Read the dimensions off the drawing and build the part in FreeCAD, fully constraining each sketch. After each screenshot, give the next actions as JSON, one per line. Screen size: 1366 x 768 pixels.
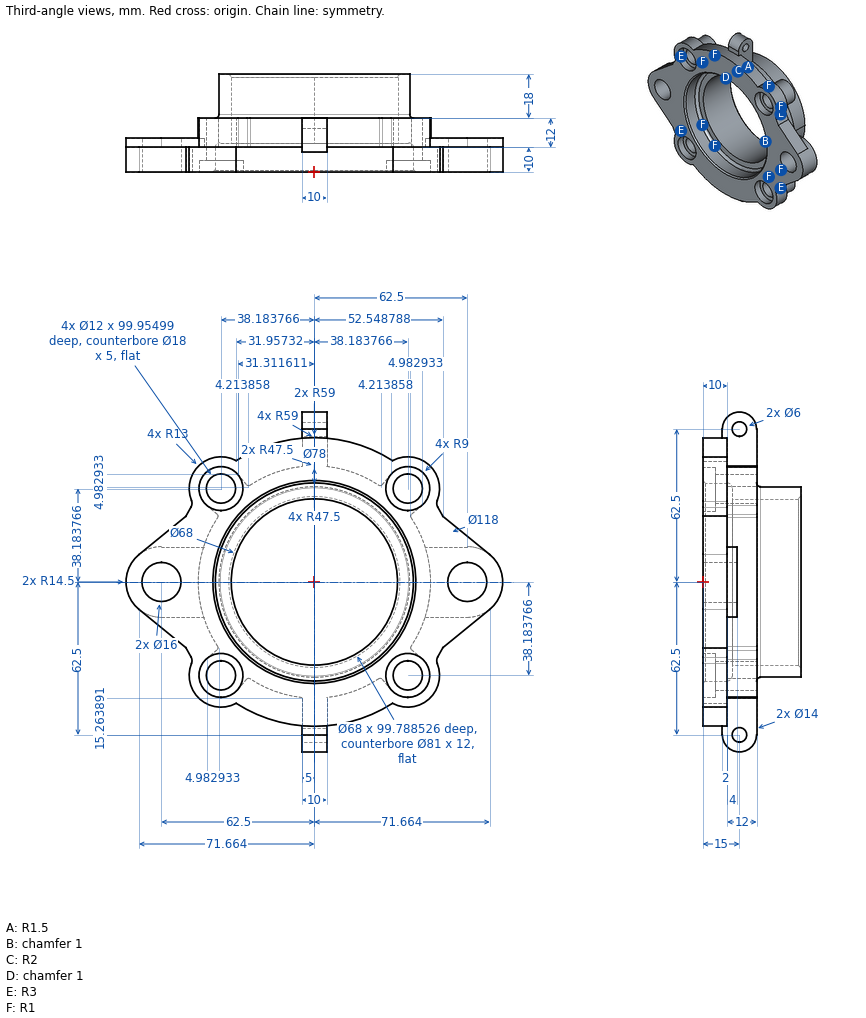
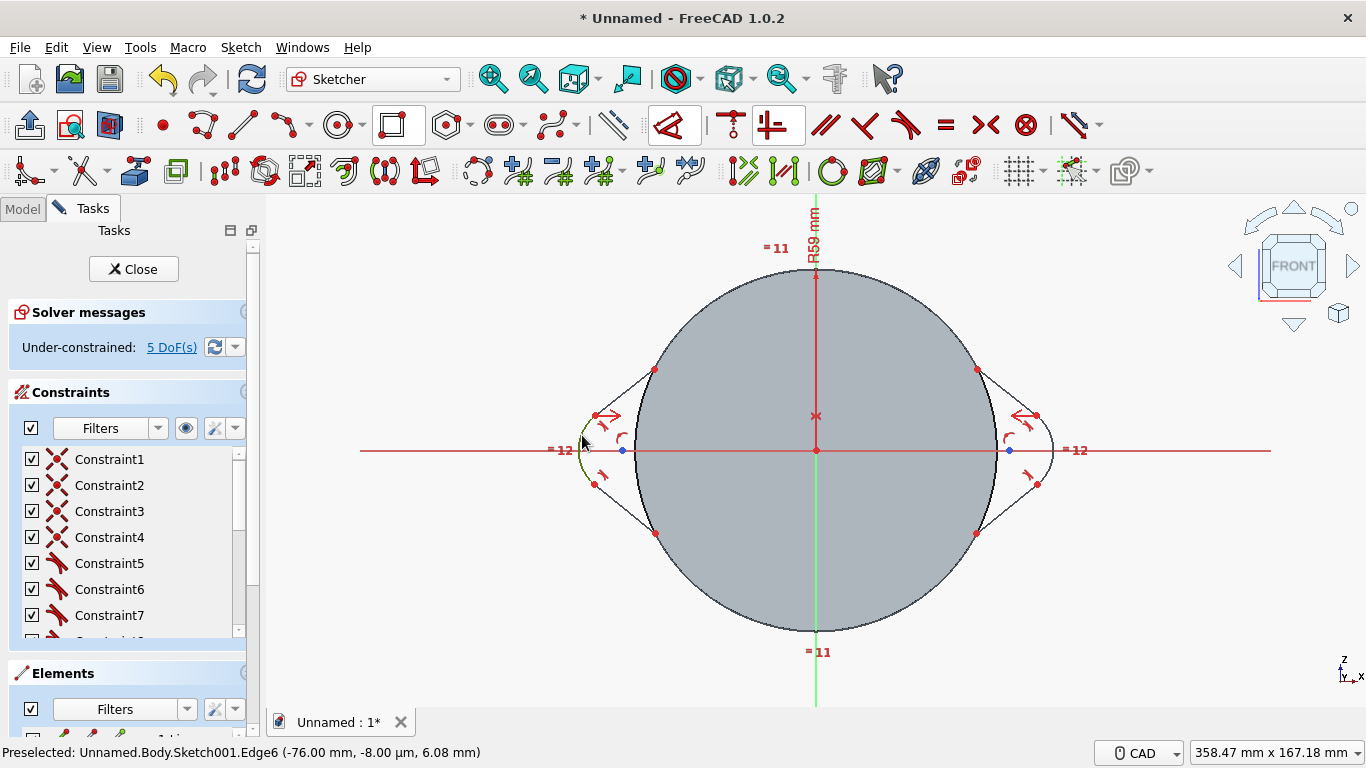
{"action": "left_click", "coordinate": [696, 126]}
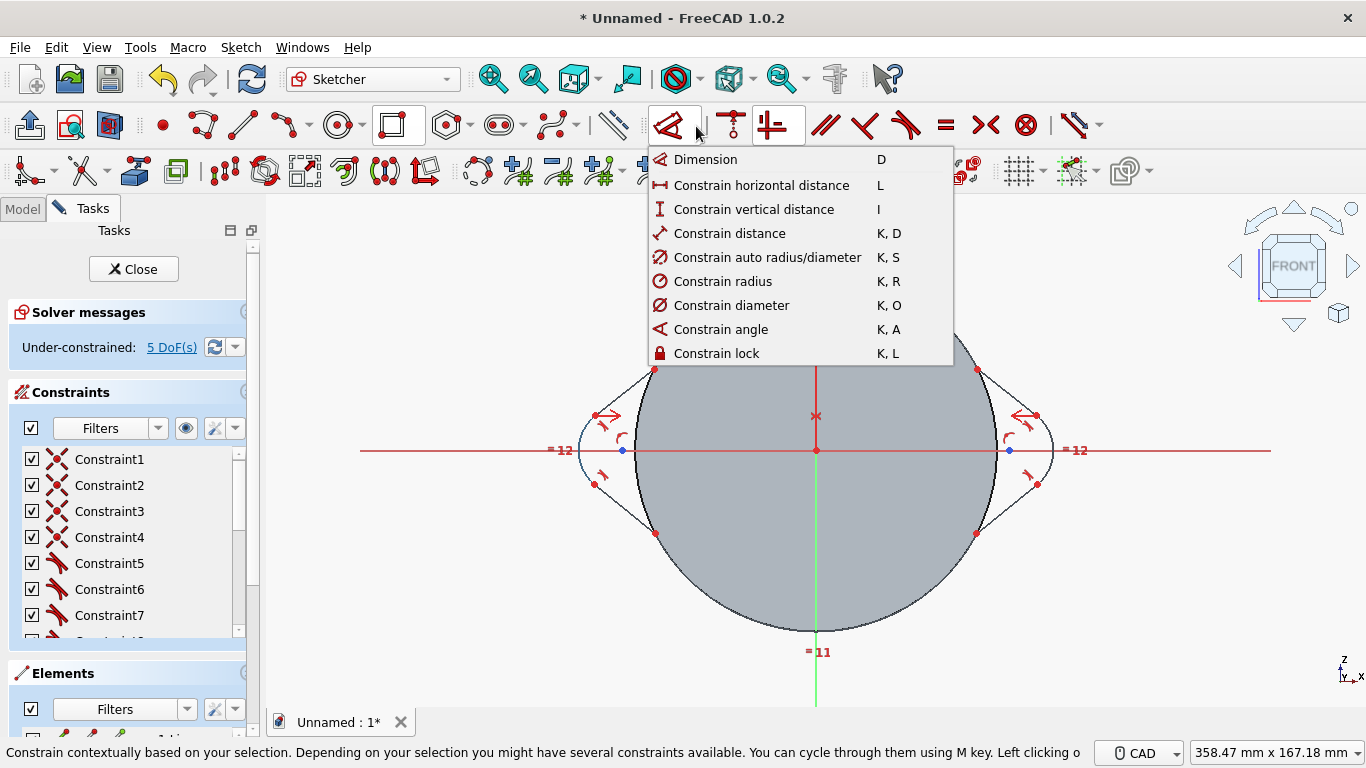
{"action": "left_click", "coordinate": [801, 281]}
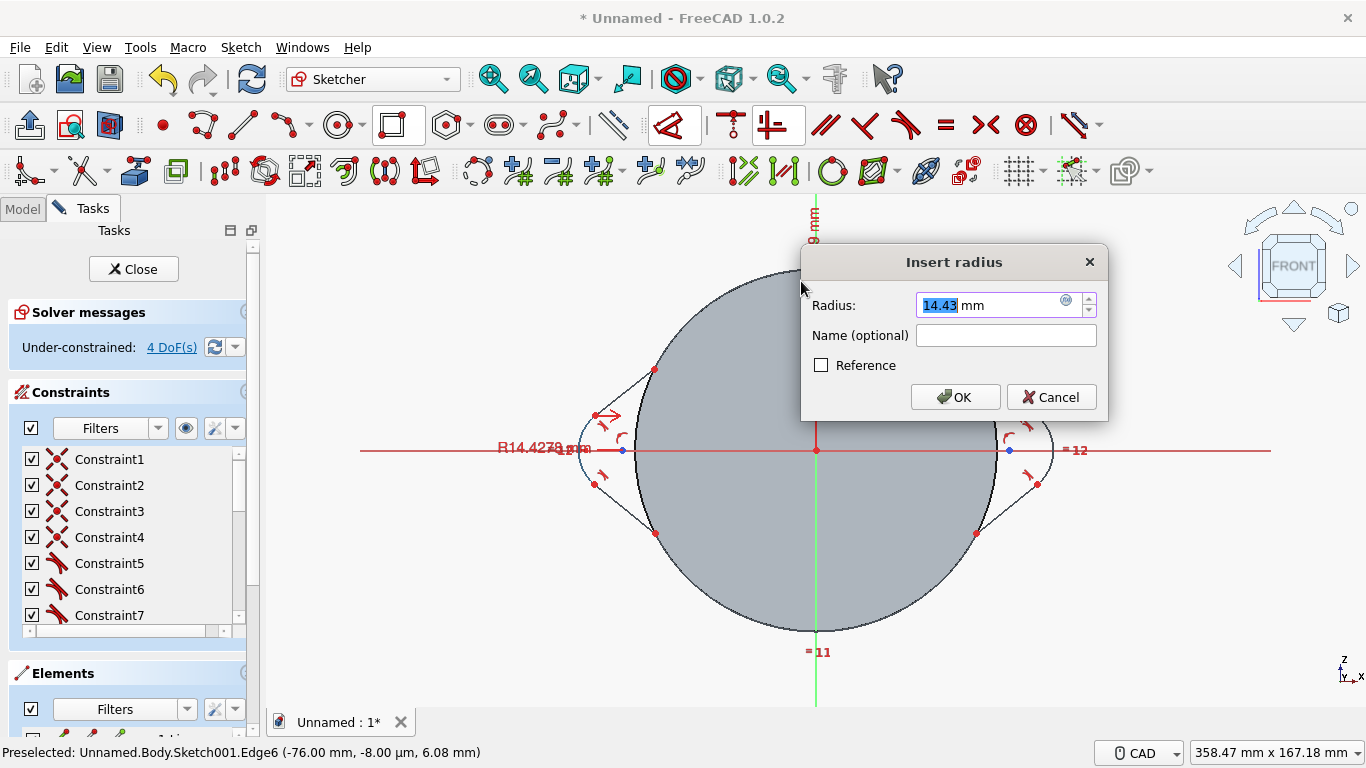
{"action": "type", "text": "14.5"}
{"action": "key", "text": "Return"}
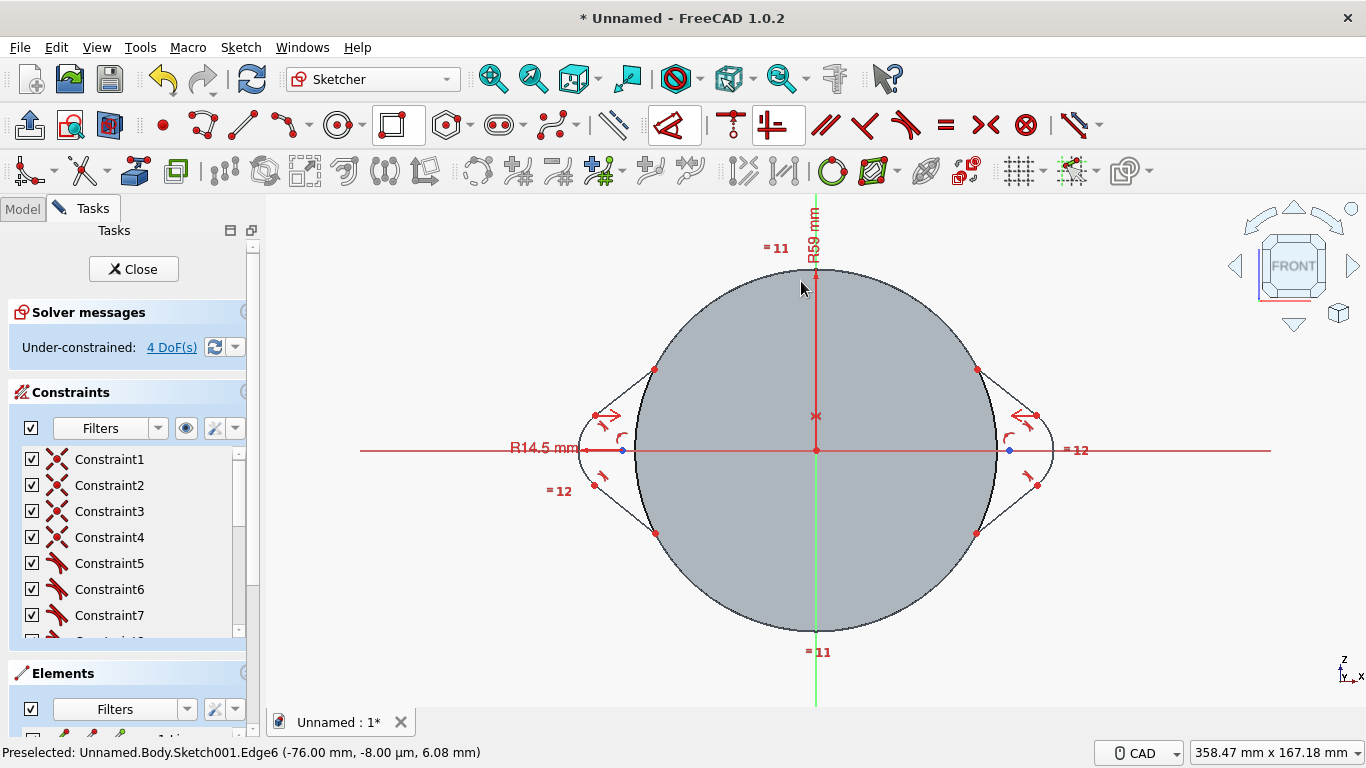
{"action": "left_click", "coordinate": [623, 450]}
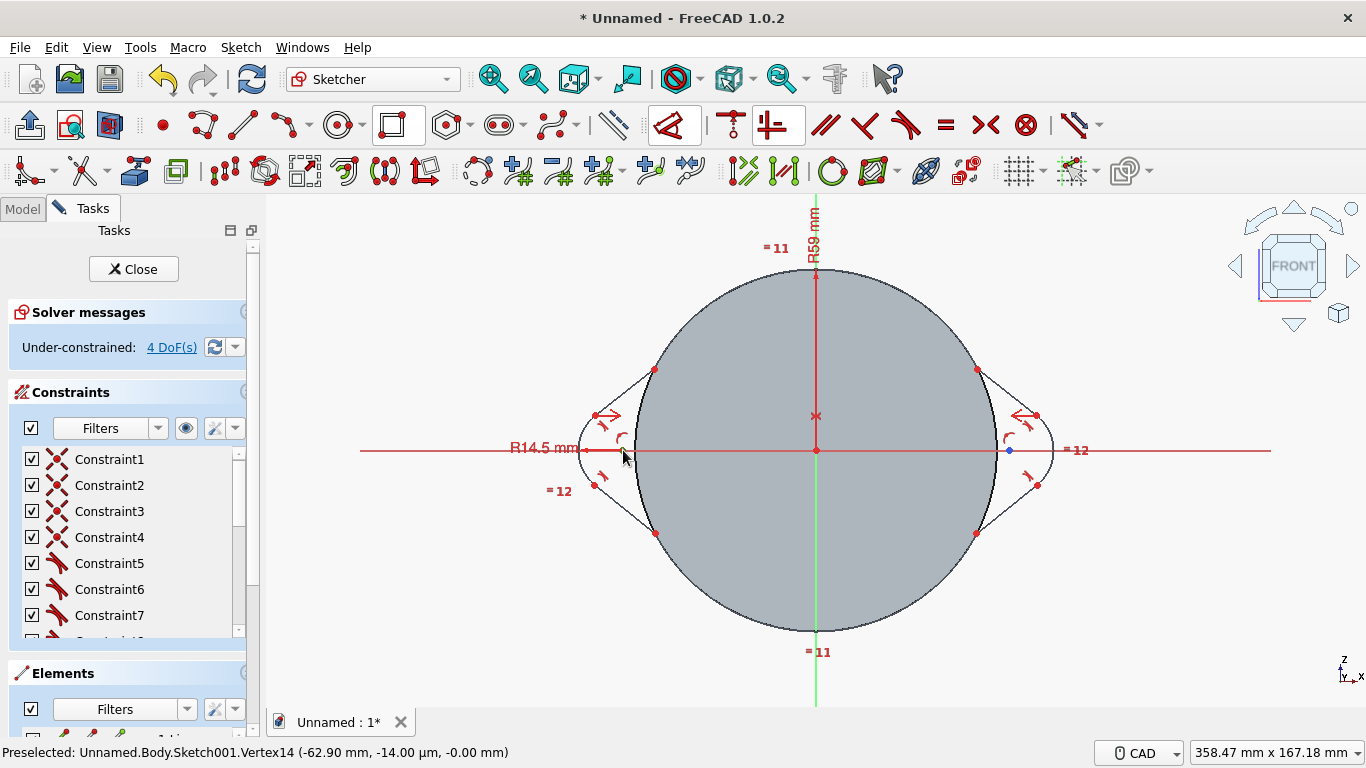
{"action": "left_click", "coordinate": [696, 126]}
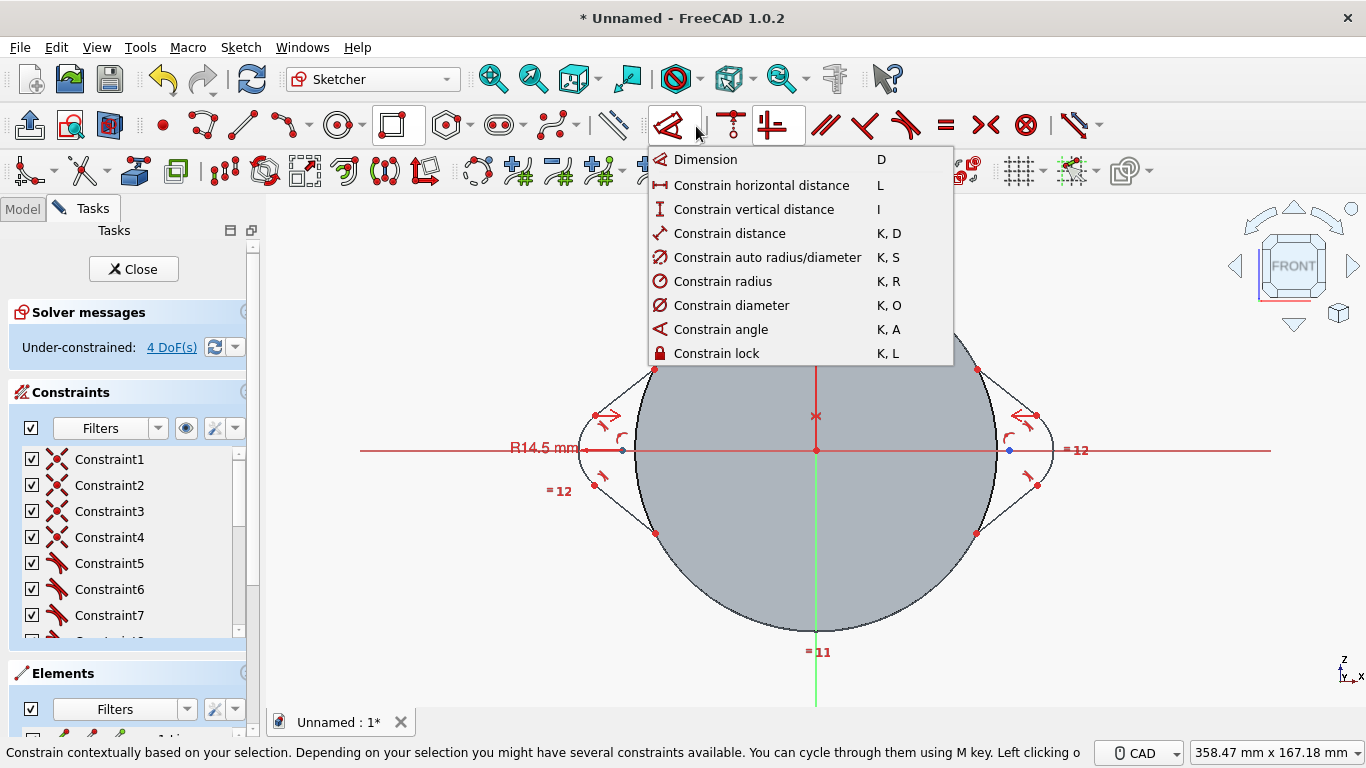
{"action": "left_click", "coordinate": [801, 185]}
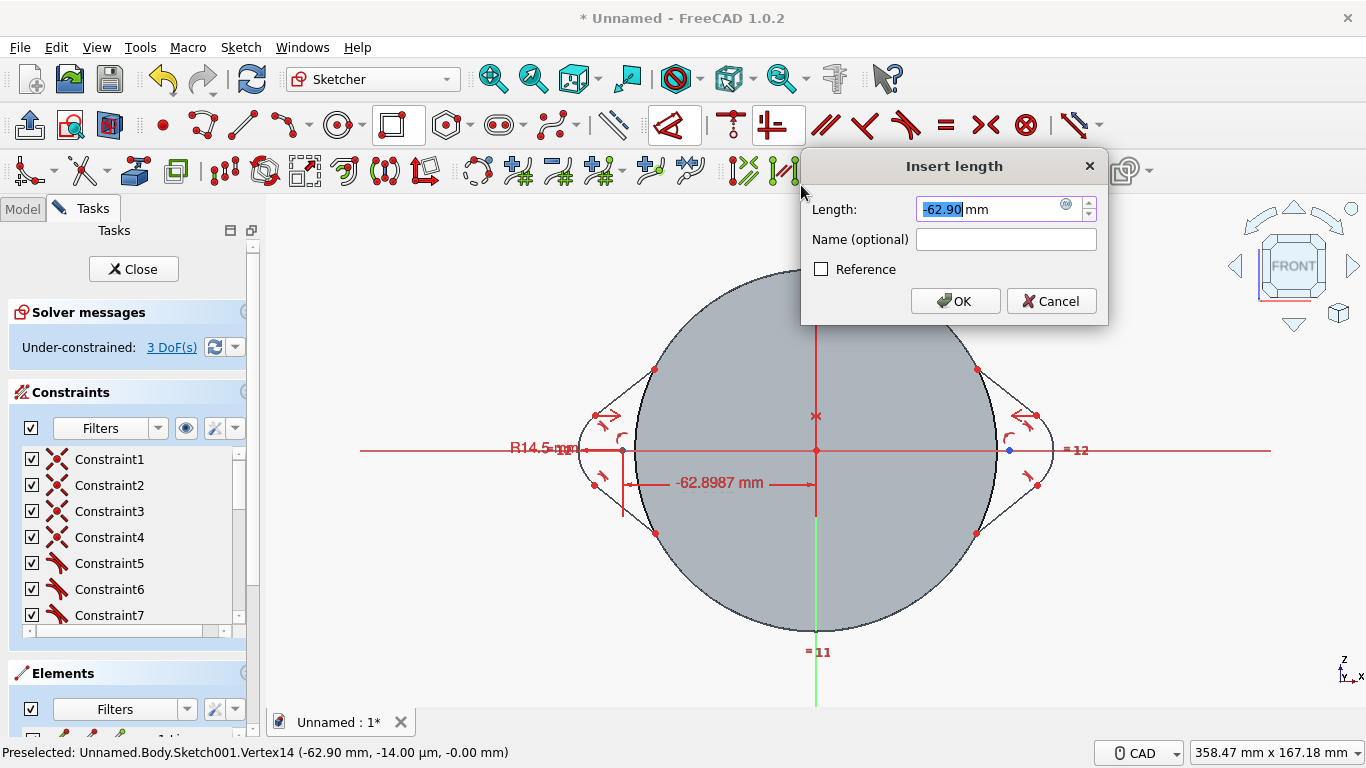
{"action": "type", "text": "-62.5"}
{"action": "key", "text": "Return"}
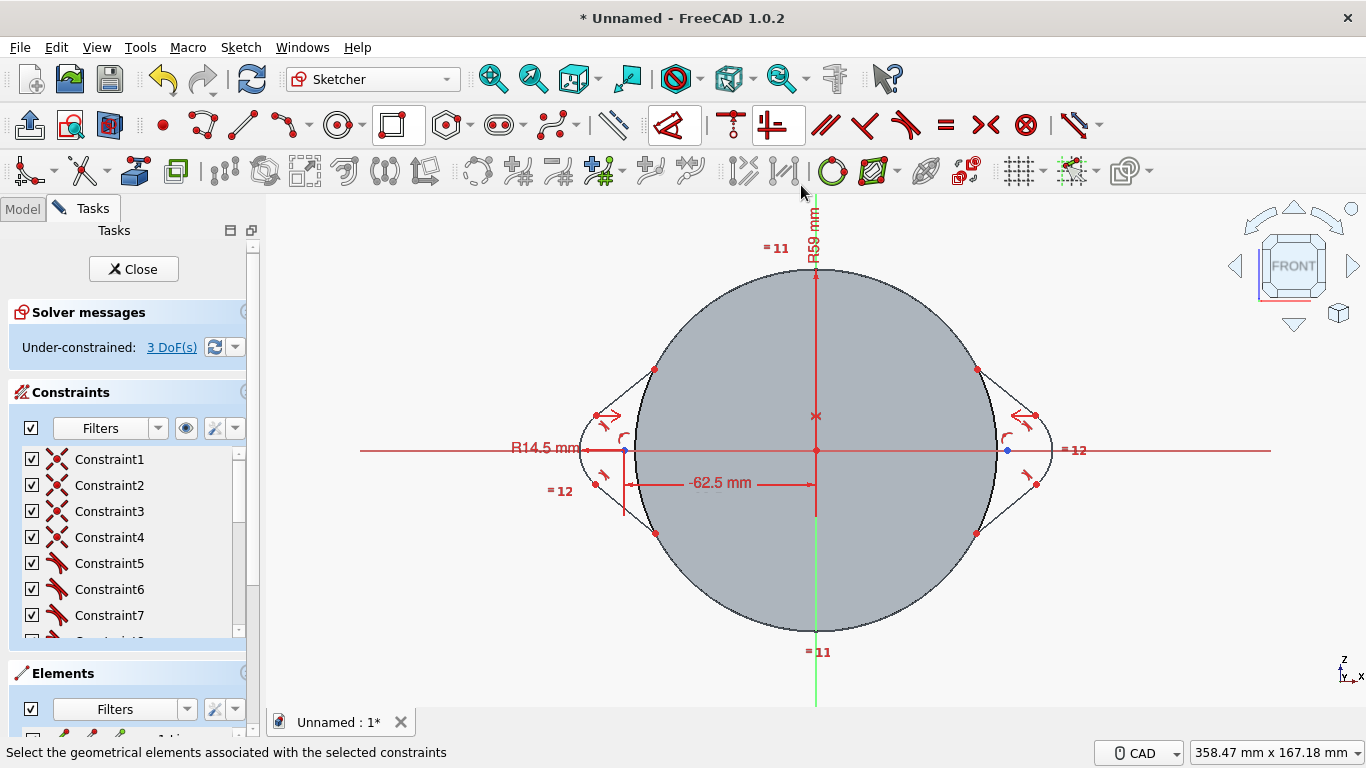
{"action": "left_click", "coordinate": [596, 485]}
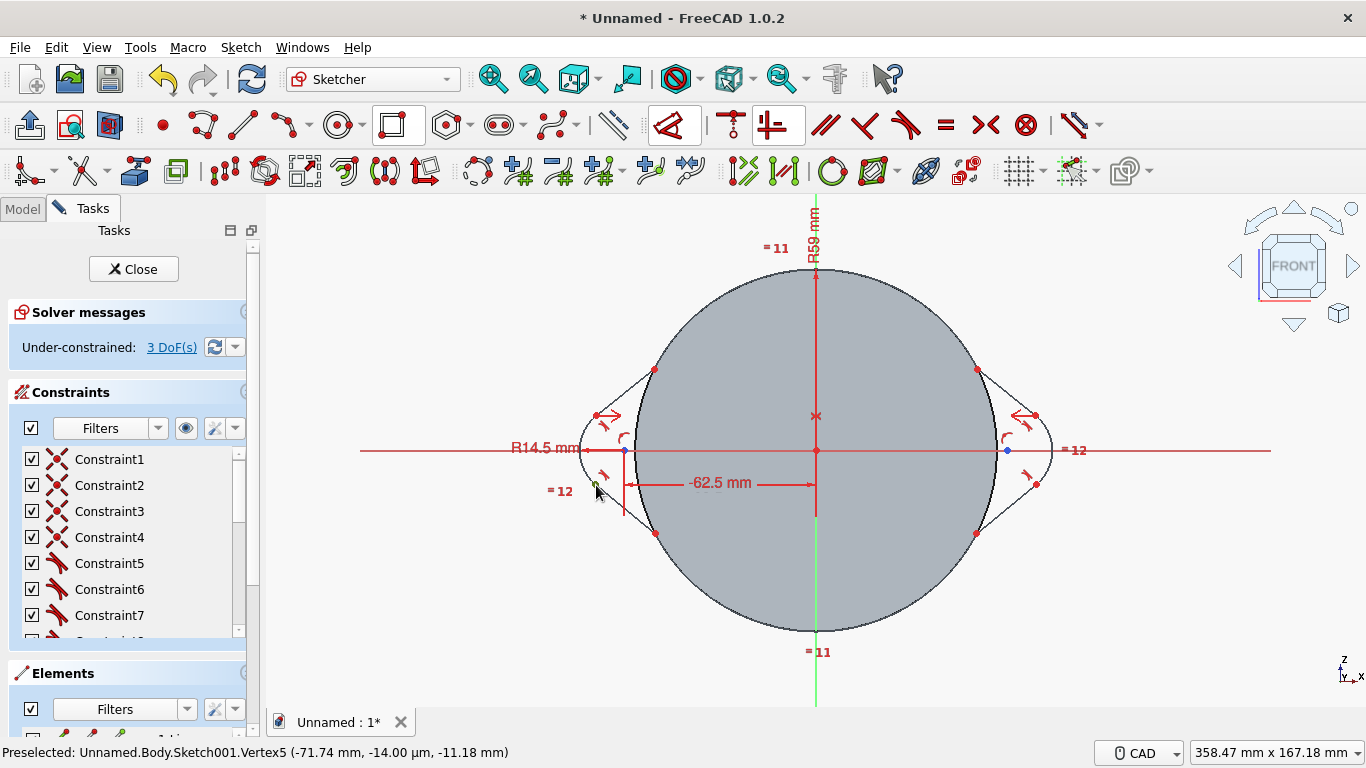
{"action": "key", "text": "l"}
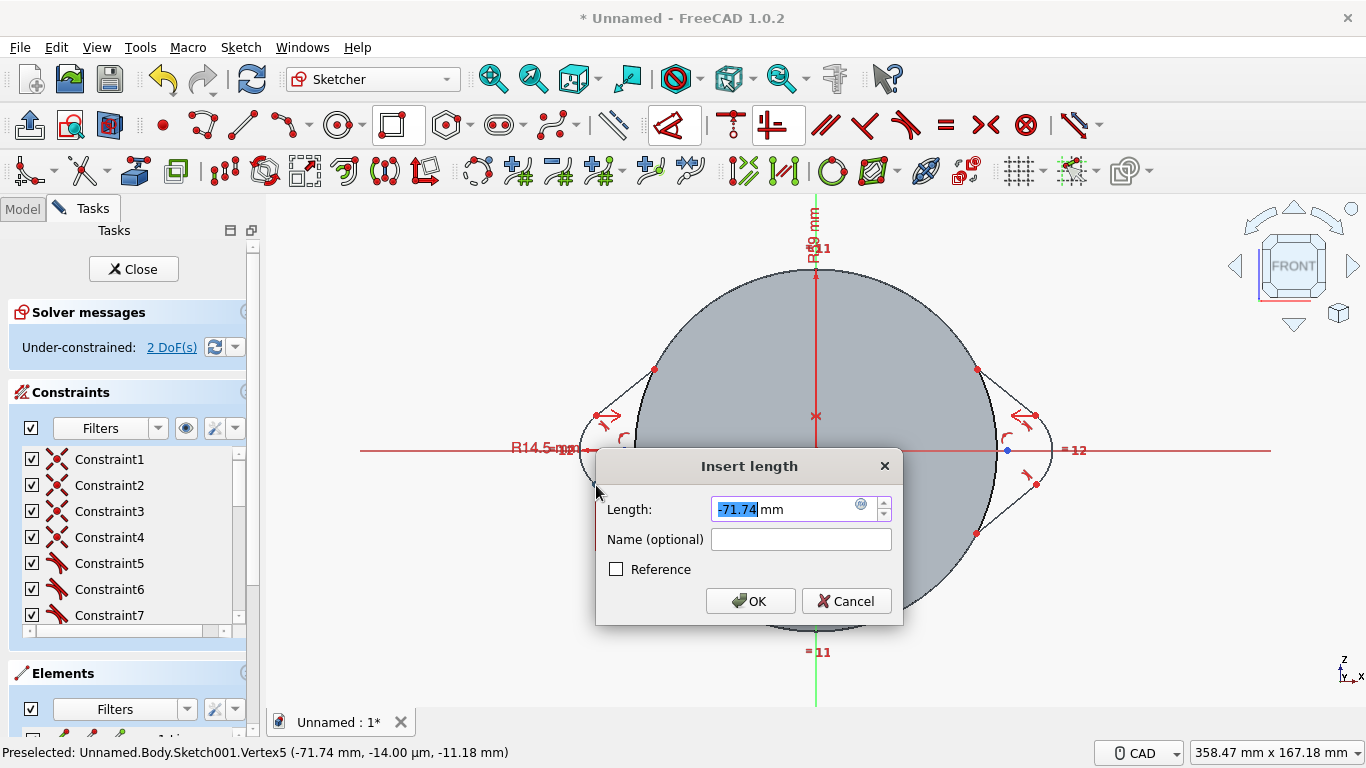
{"action": "type", "text": "-71.664"}
{"action": "key", "text": "Return"}